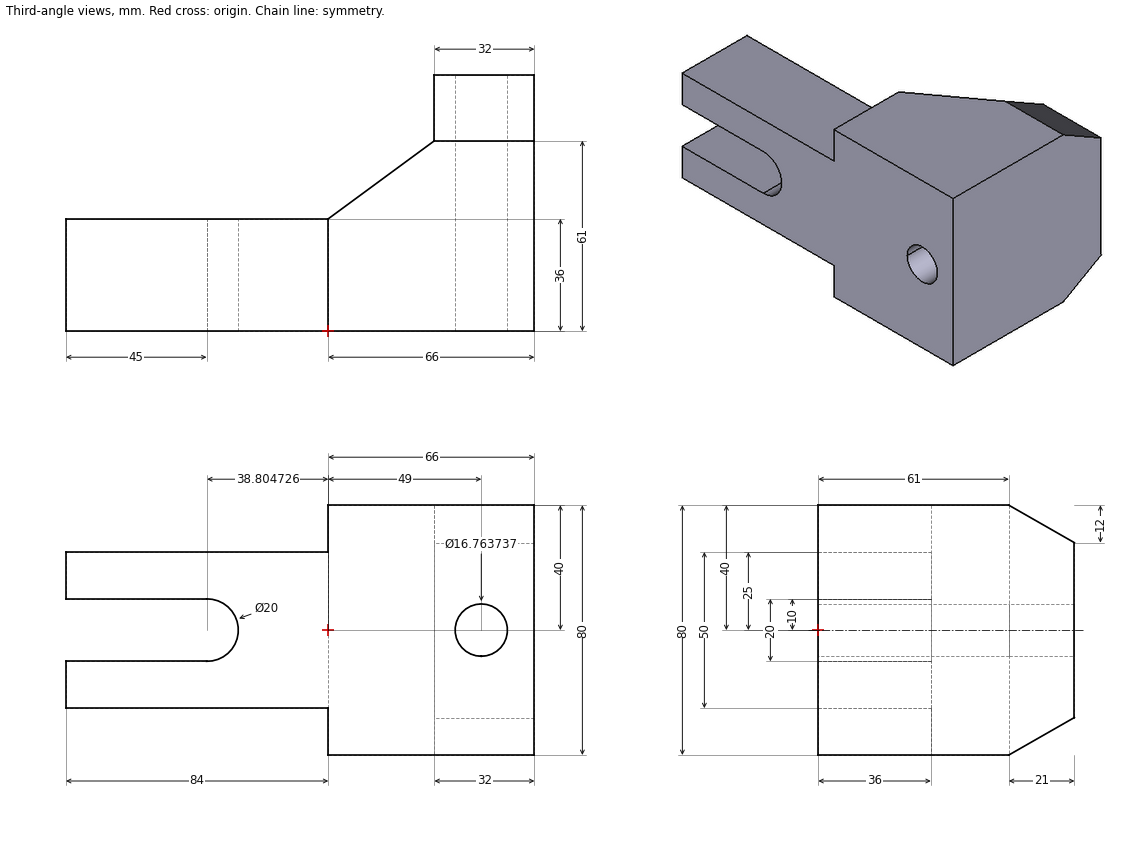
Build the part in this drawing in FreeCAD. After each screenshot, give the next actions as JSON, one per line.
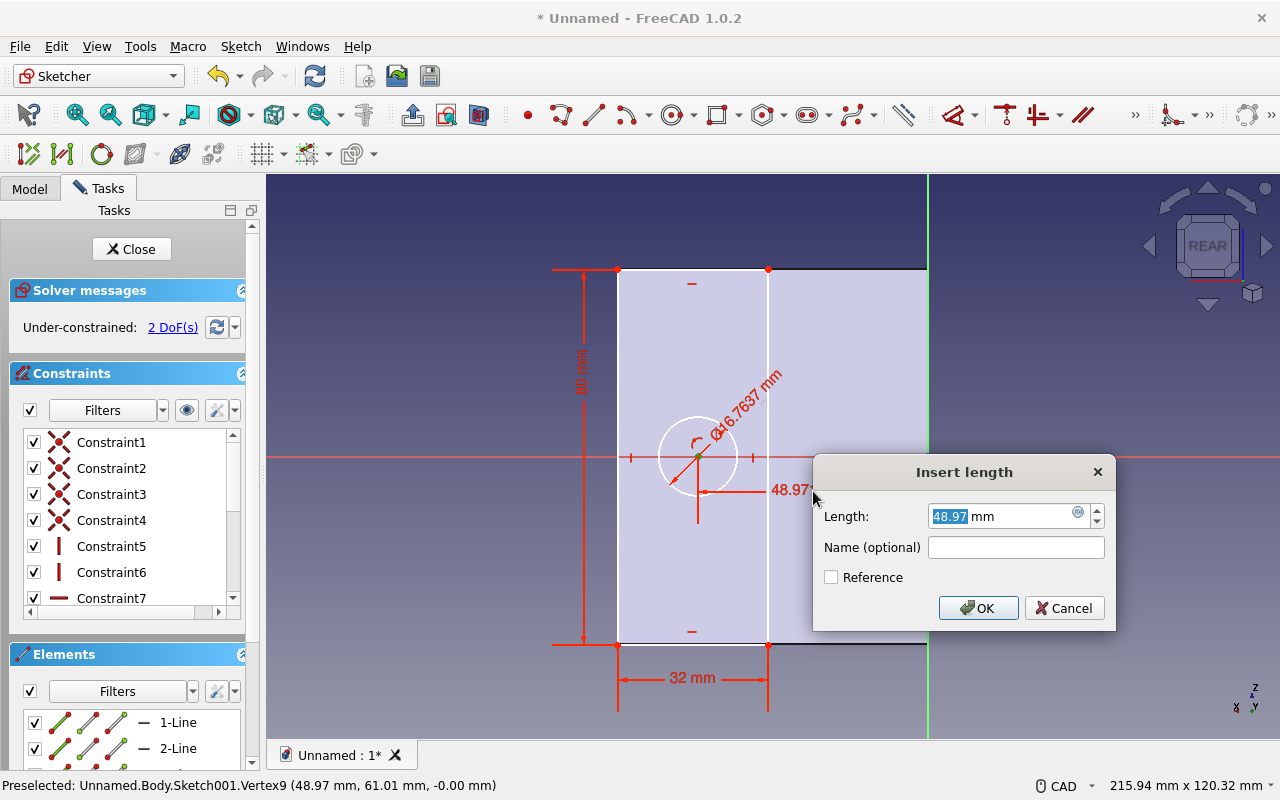
{"action": "type", "text": "49"}
{"action": "key", "text": "Return"}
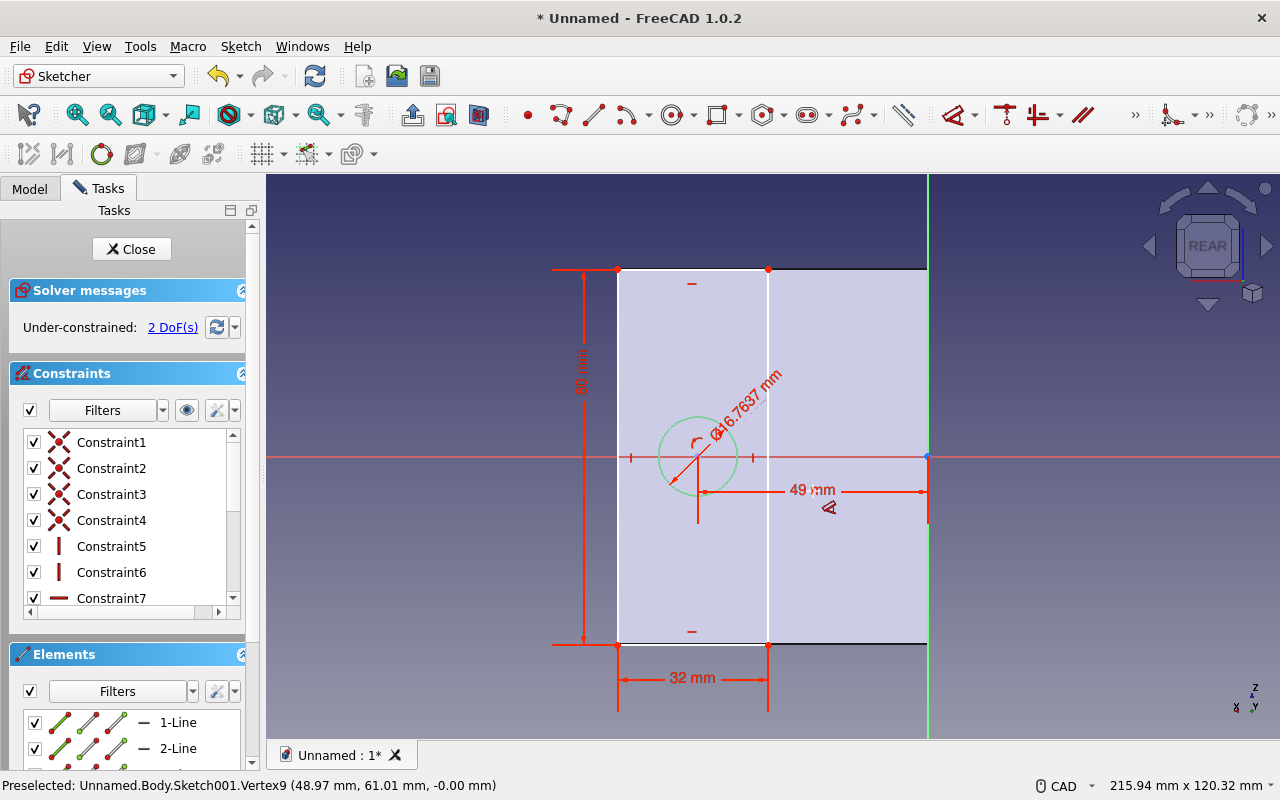
{"action": "left_click", "coordinate": [618, 270]}
{"action": "left_click", "coordinate": [773, 236]}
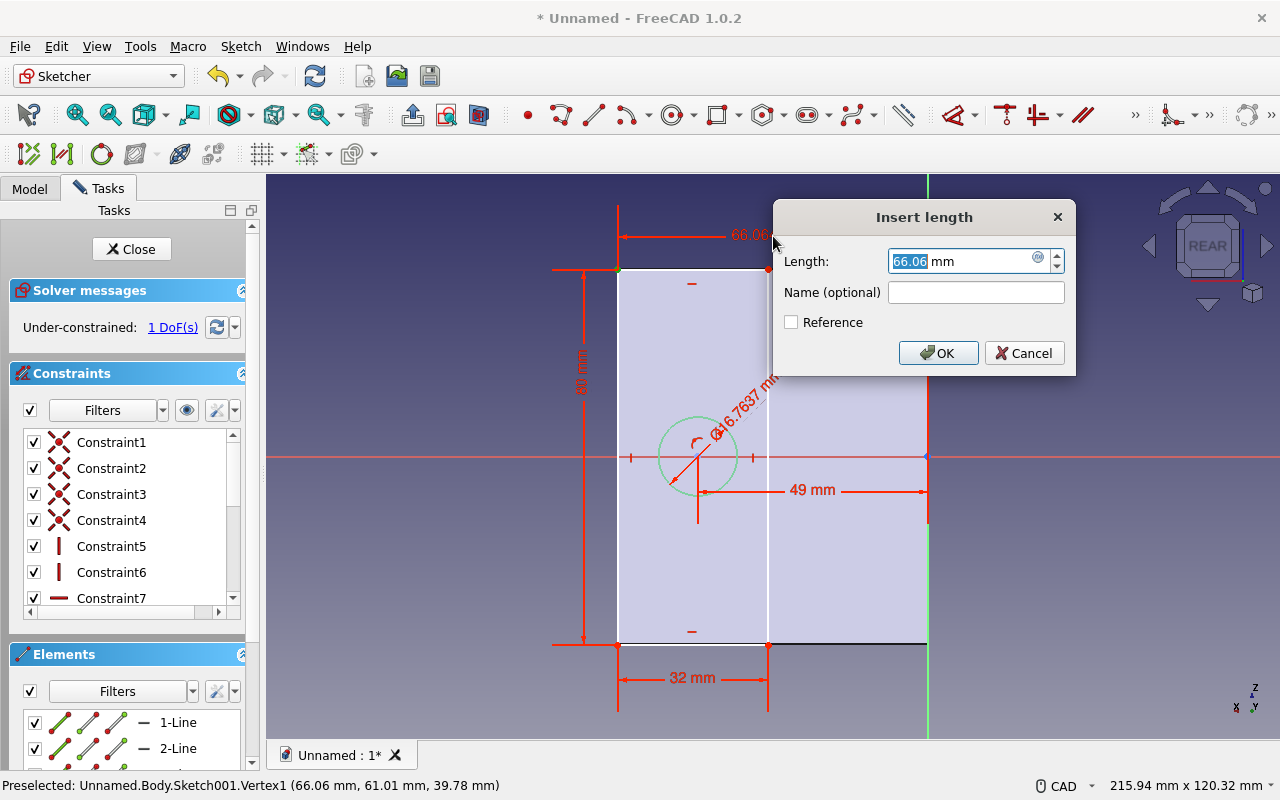
{"action": "type", "text": "66"}
{"action": "key", "text": "Return"}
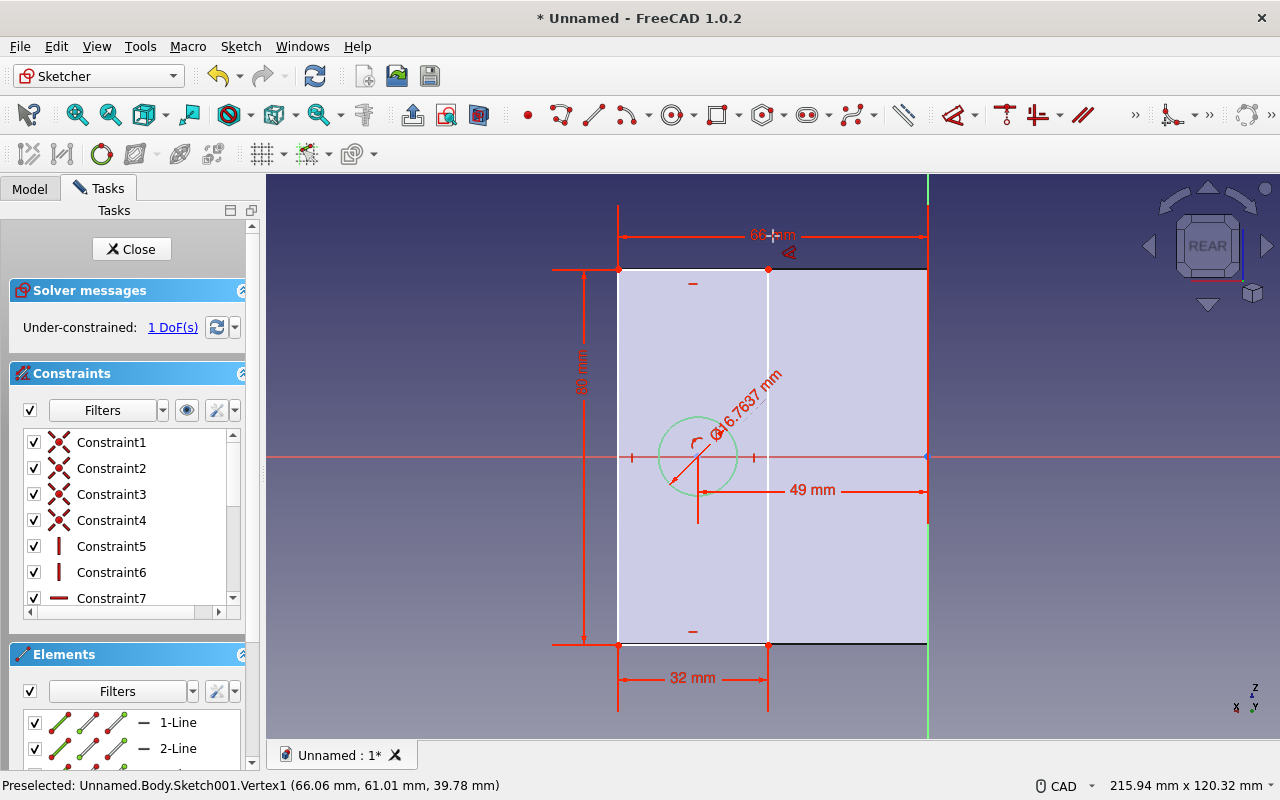
{"action": "left_click", "coordinate": [618, 270]}
{"action": "left_click", "coordinate": [962, 363]}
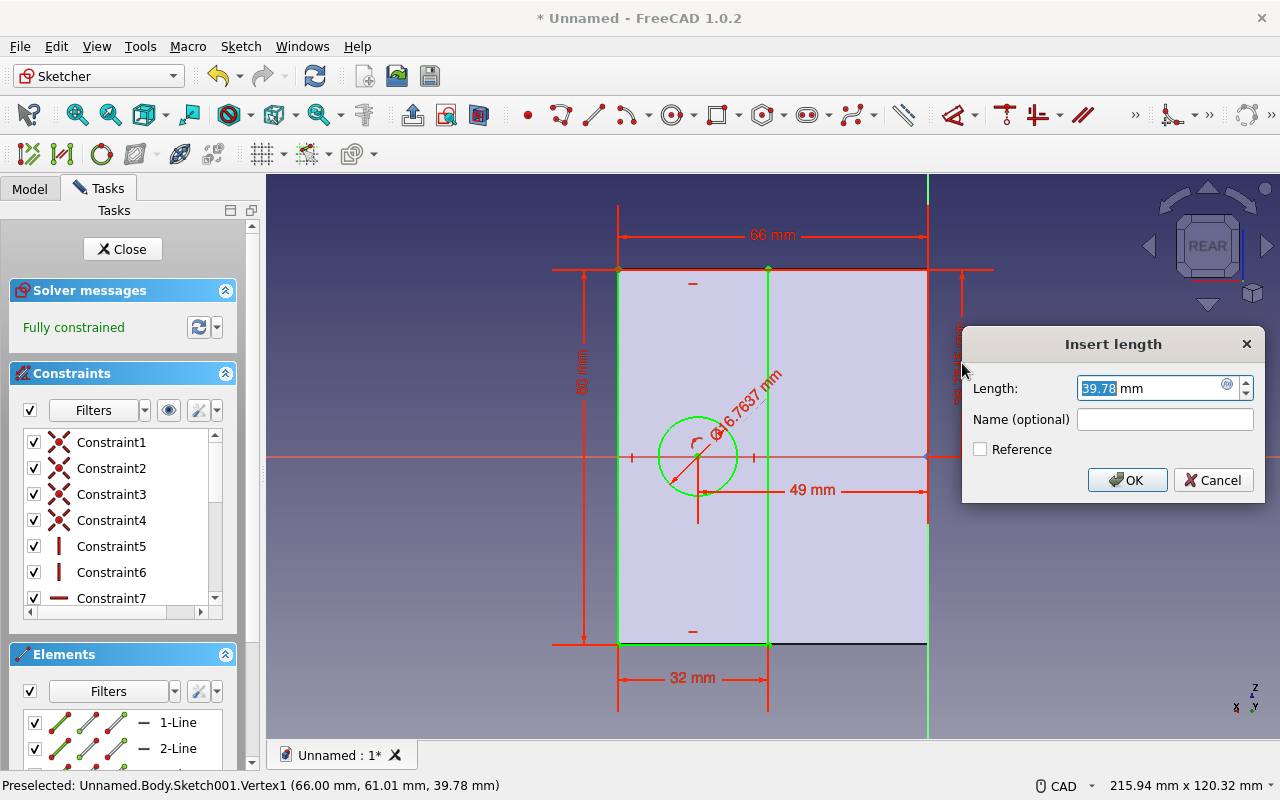
{"action": "type", "text": "40"}
{"action": "key", "text": "Return"}
{"action": "key", "text": "Escape"}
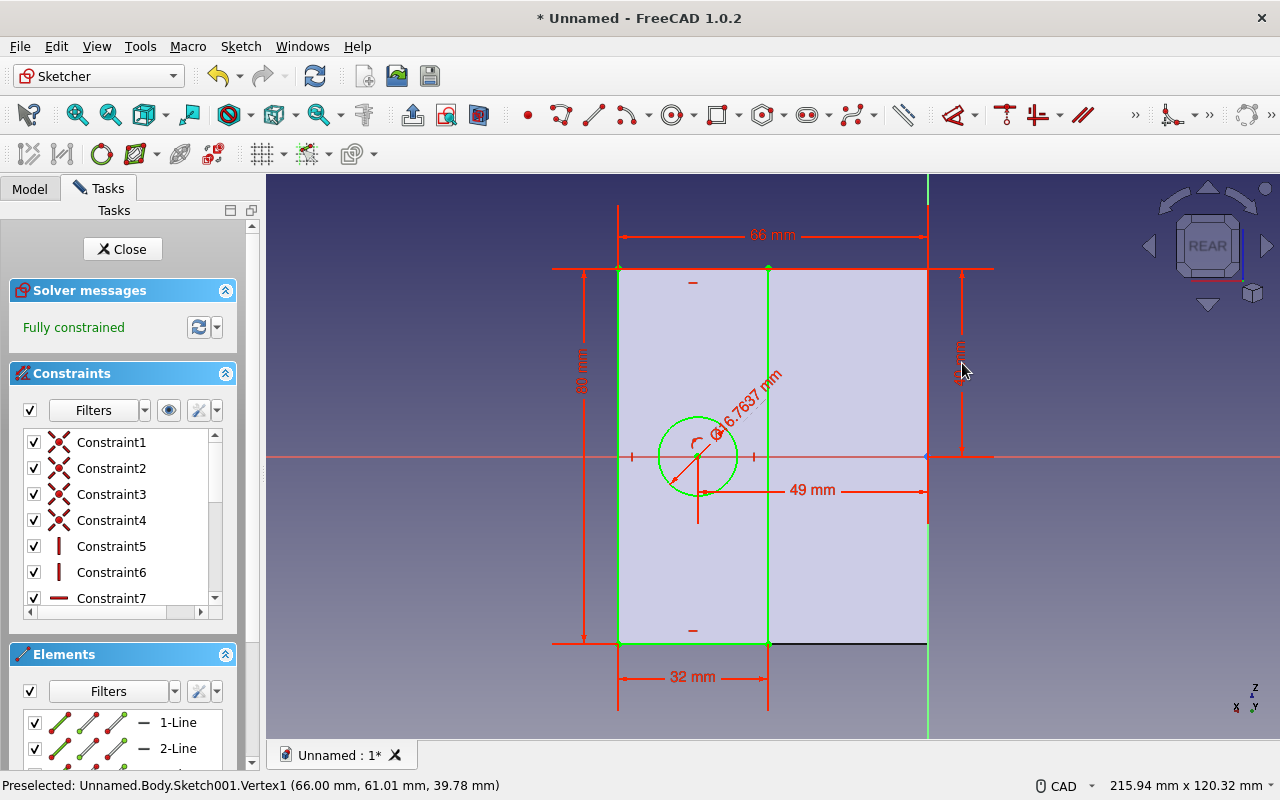
{"action": "left_click", "coordinate": [123, 249]}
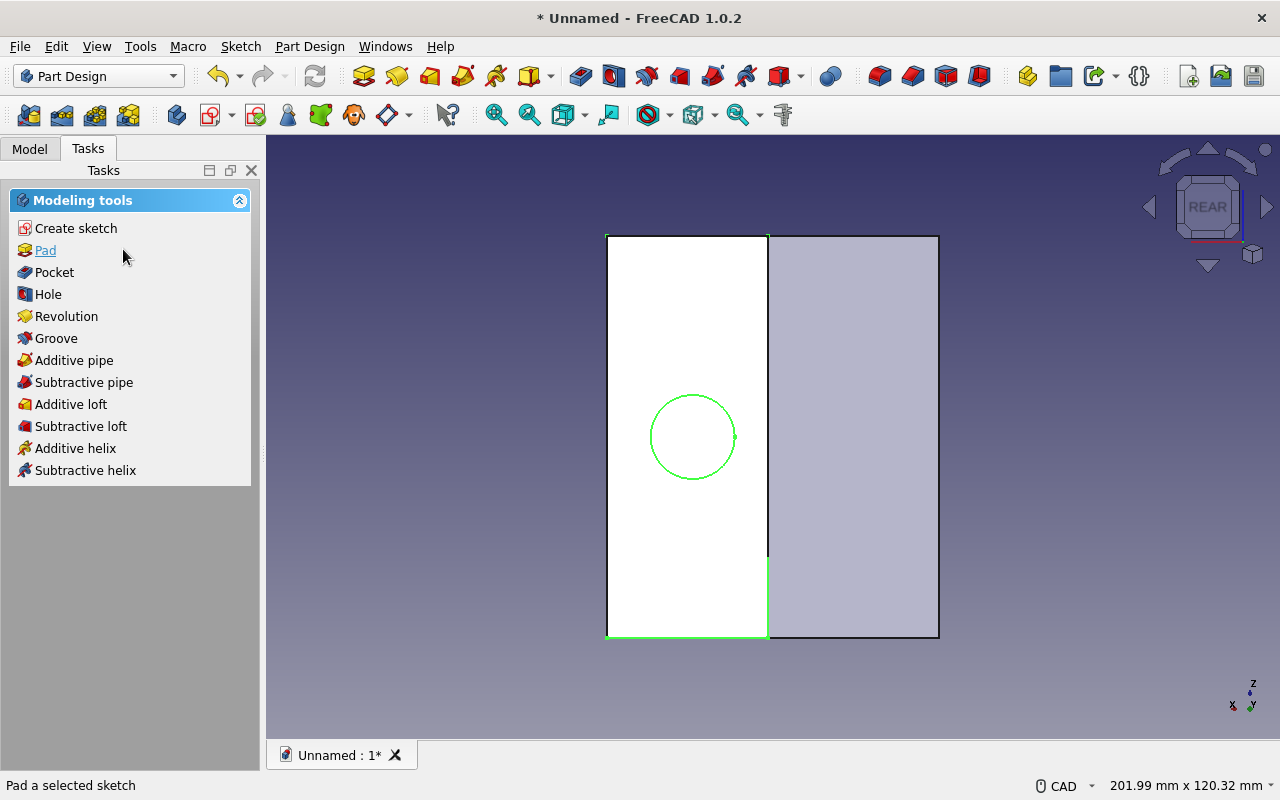
{"action": "left_click", "coordinate": [364, 76]}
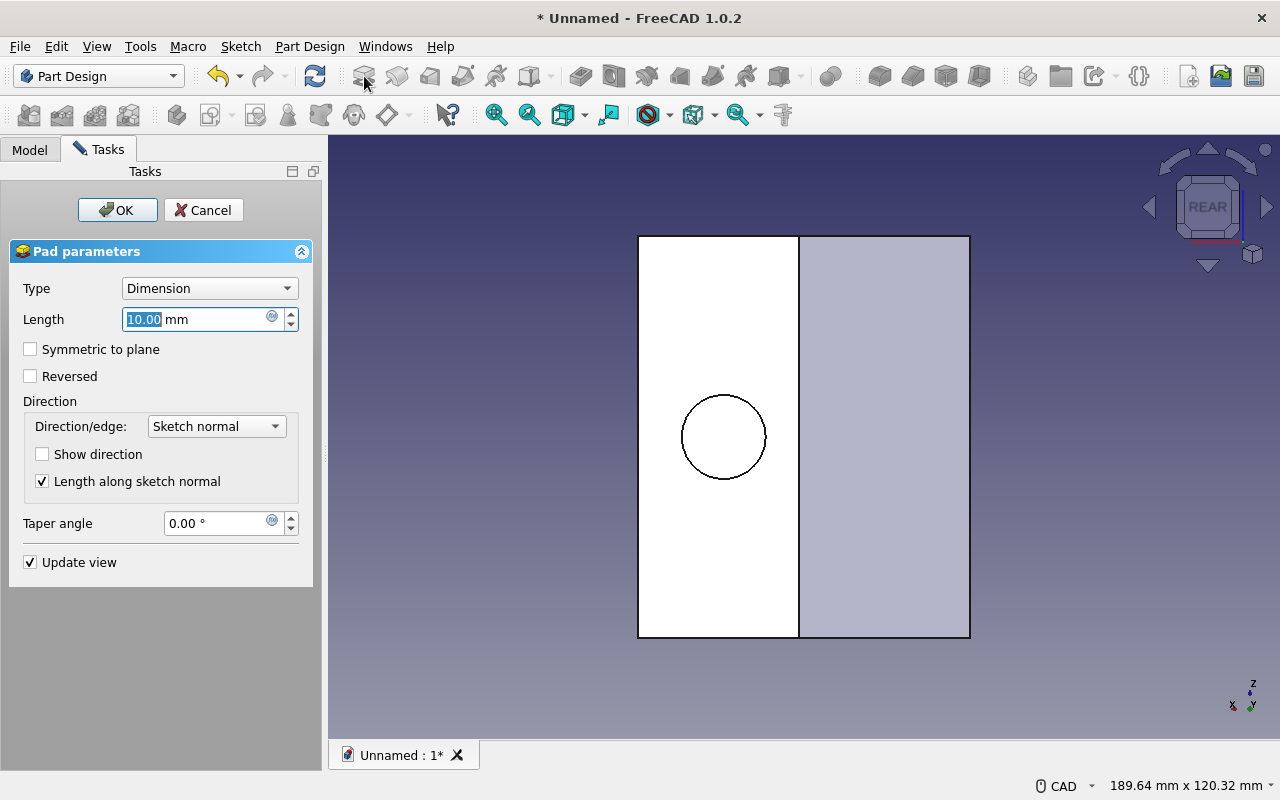
{"action": "type", "text": "21"}
{"action": "key", "text": "Tab"}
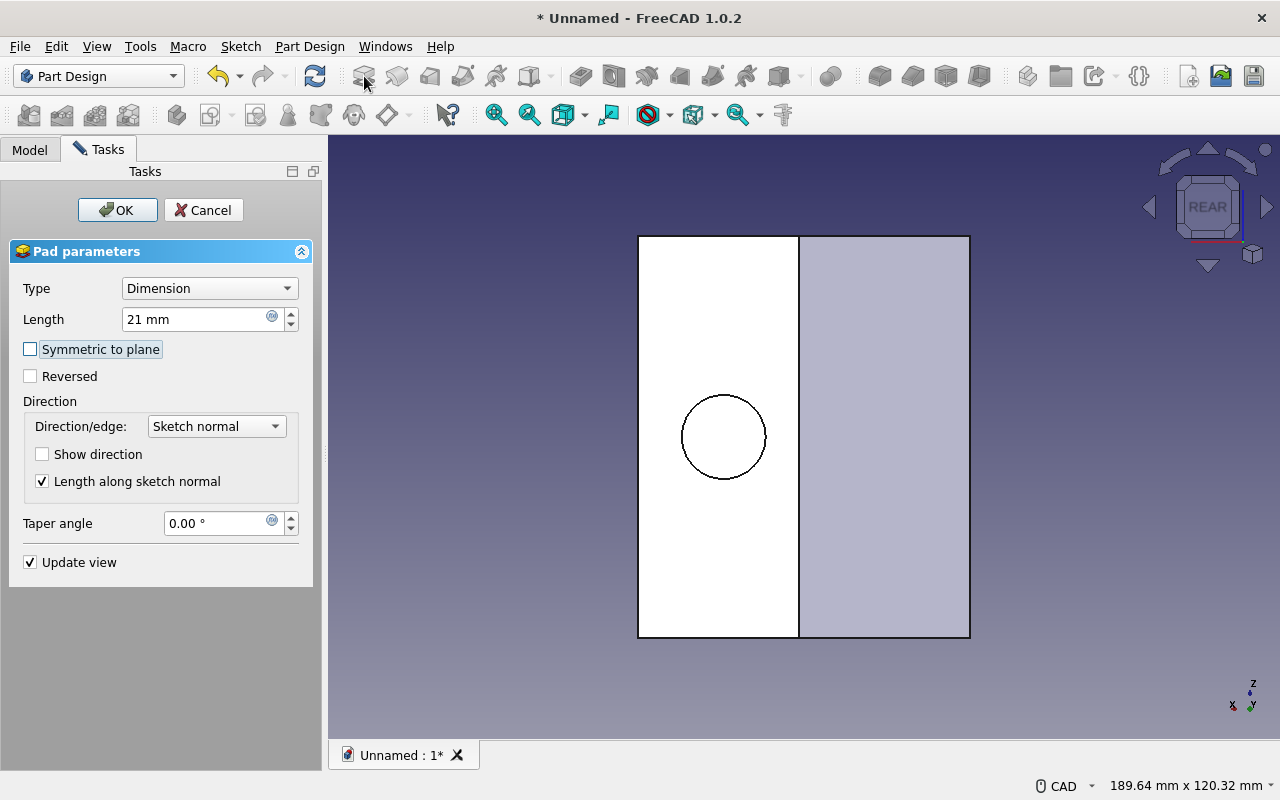
{"action": "left_click", "coordinate": [118, 210]}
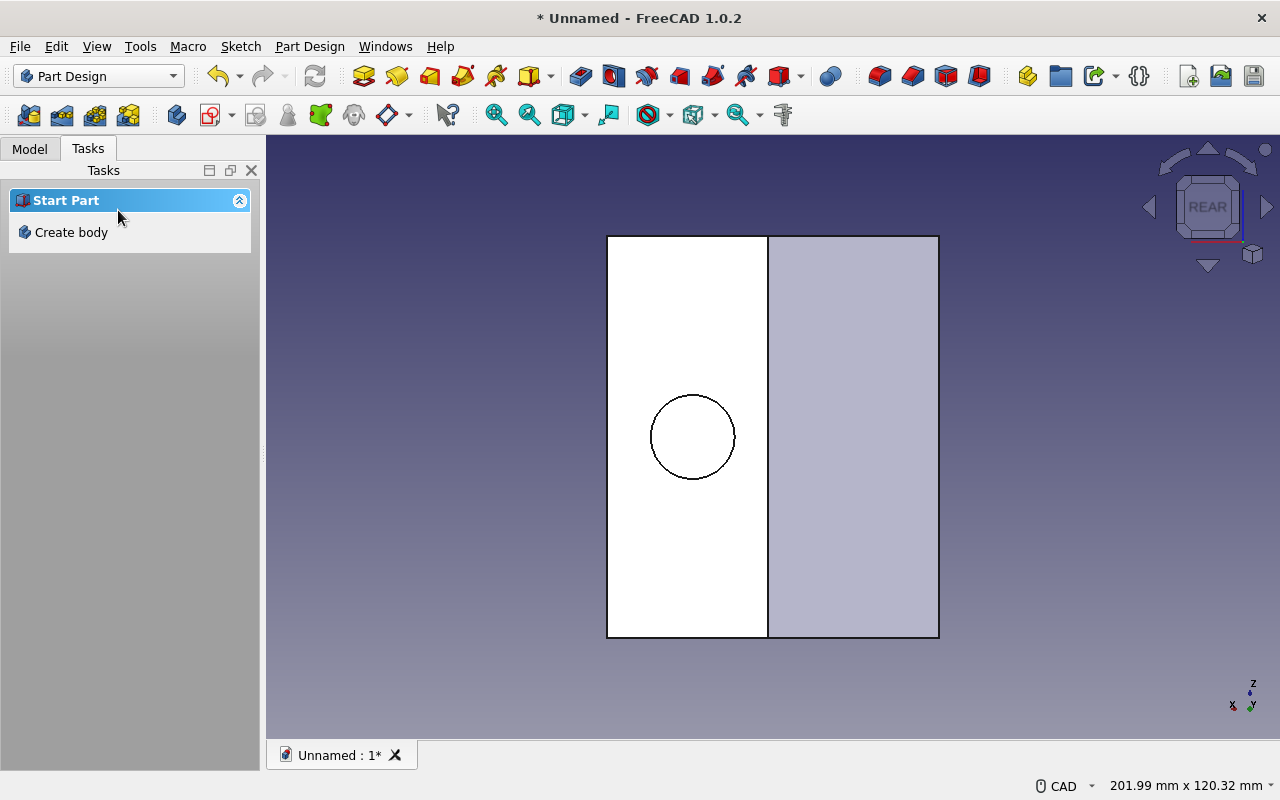
{"action": "key", "text": "0"}